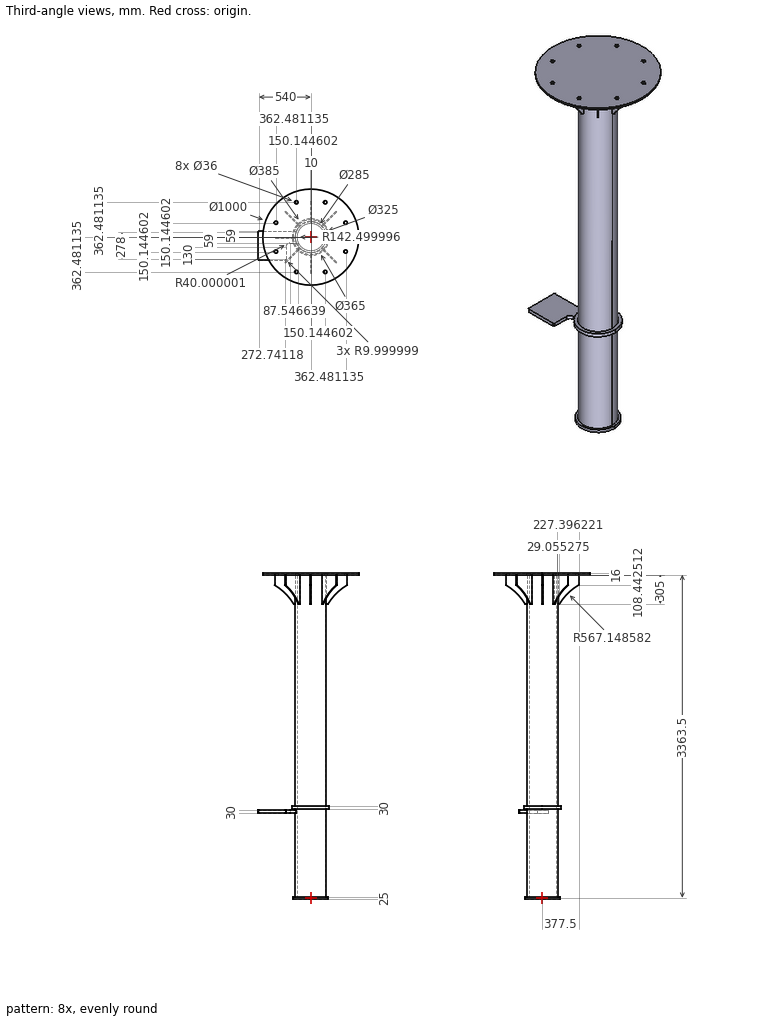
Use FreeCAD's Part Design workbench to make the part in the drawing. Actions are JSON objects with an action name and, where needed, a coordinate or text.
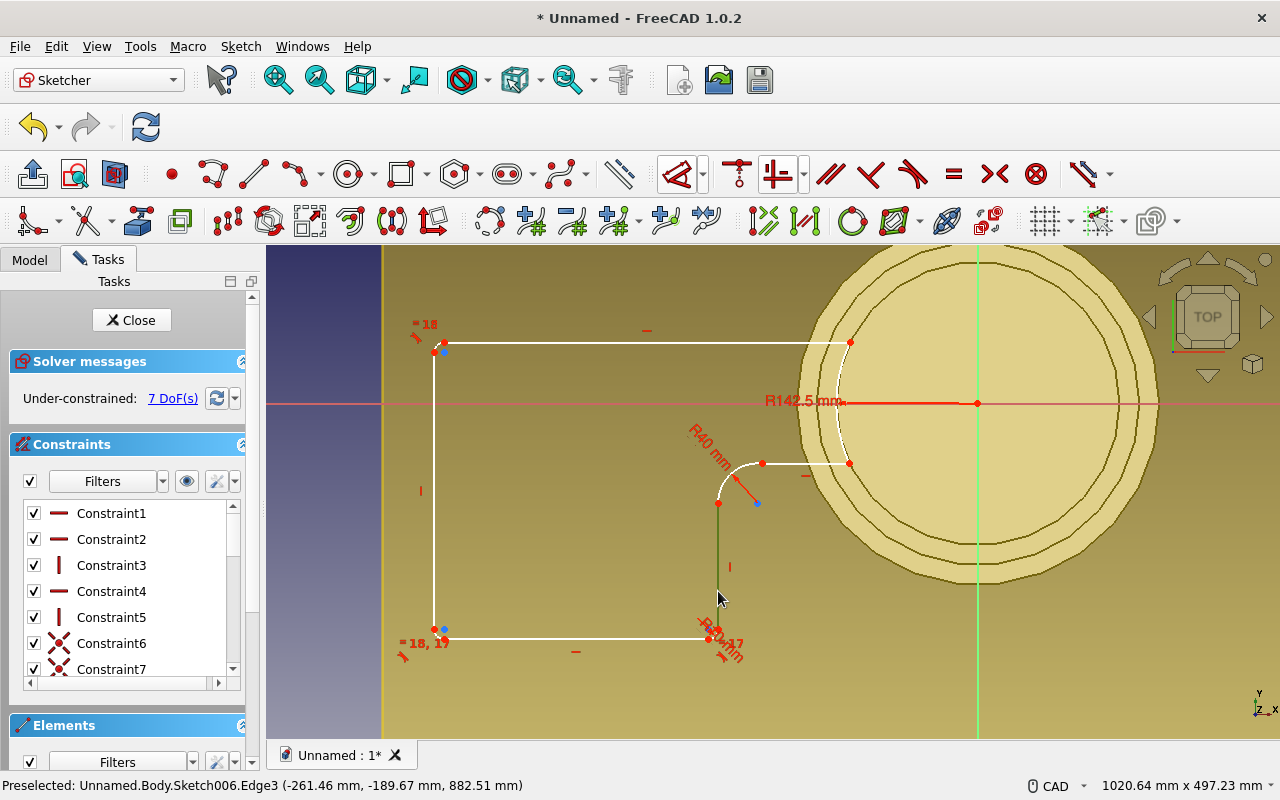
{"action": "key", "text": "i"}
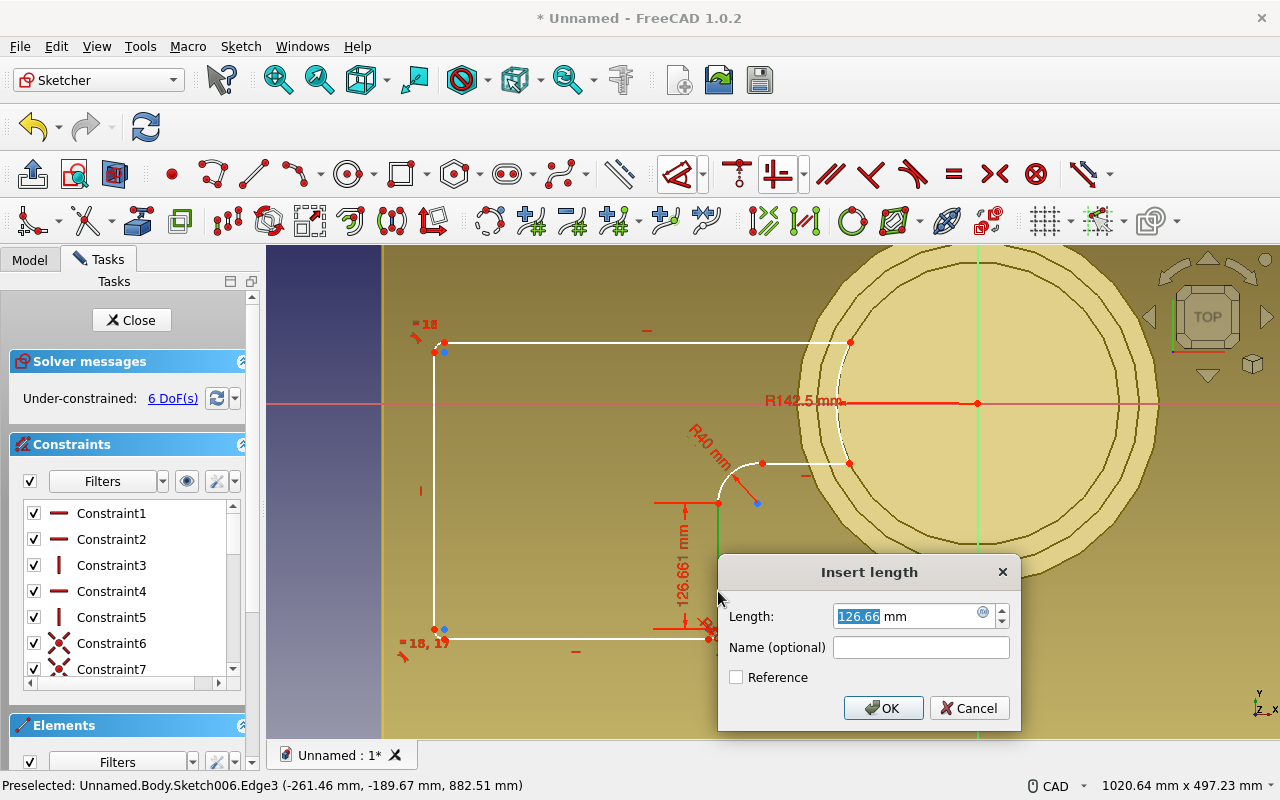
{"action": "type", "text": "130"}
{"action": "key", "text": "Return"}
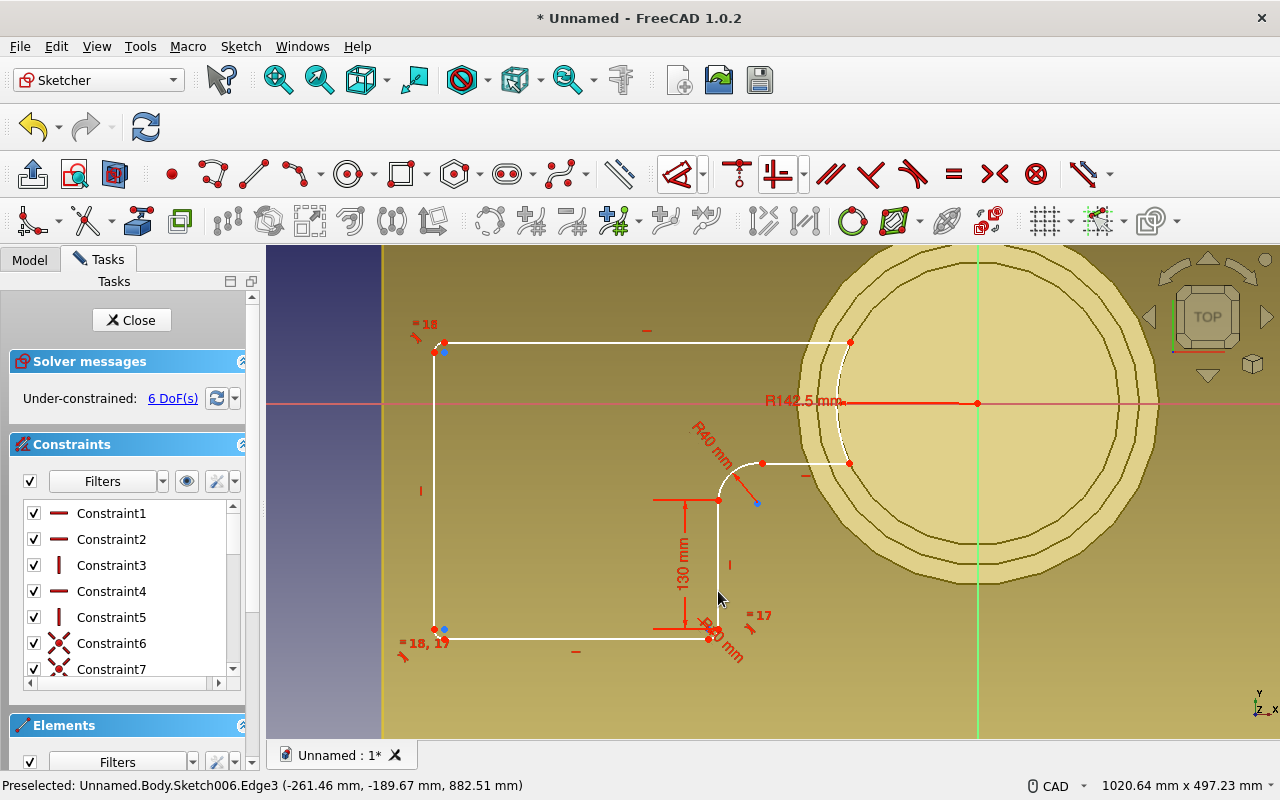
{"action": "left_click", "coordinate": [434, 546]}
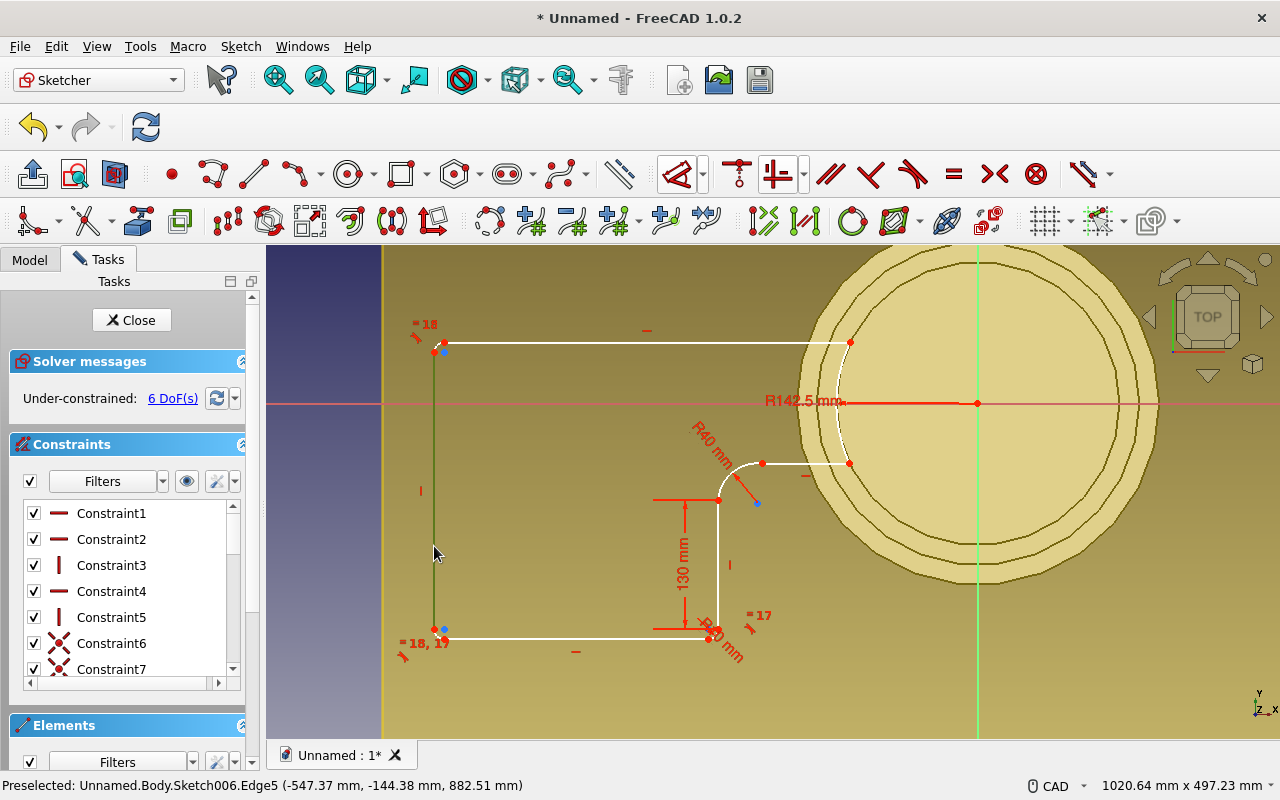
{"action": "left_click", "coordinate": [702, 174]}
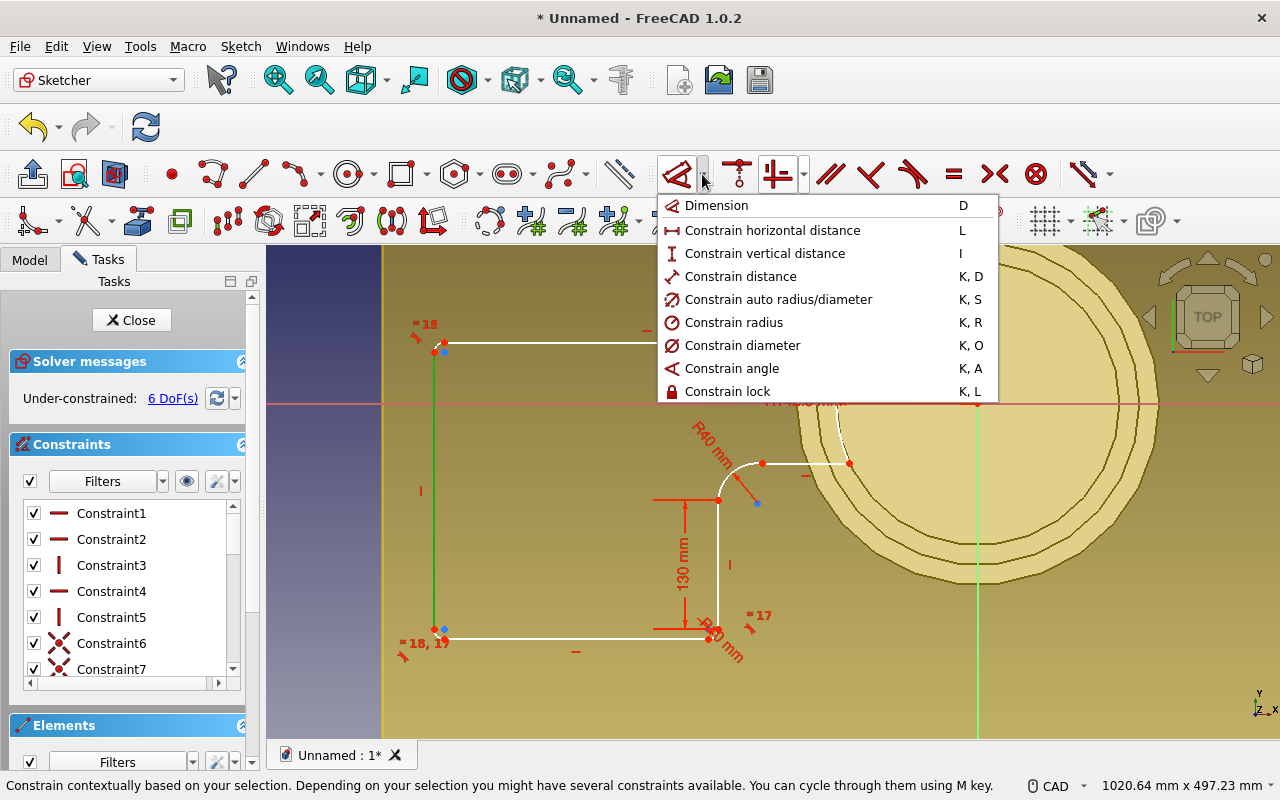
{"action": "left_click", "coordinate": [828, 254]}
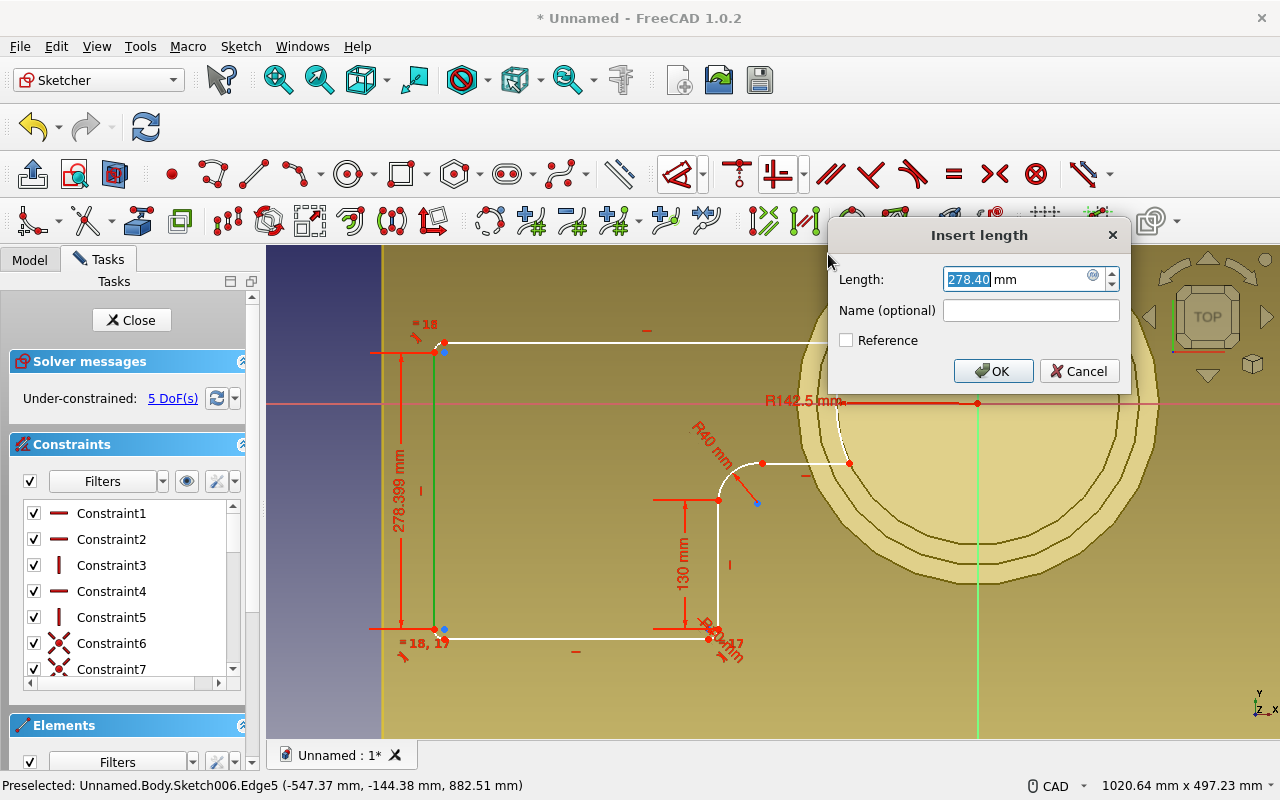
{"action": "type", "text": "278"}
{"action": "key", "text": "Return"}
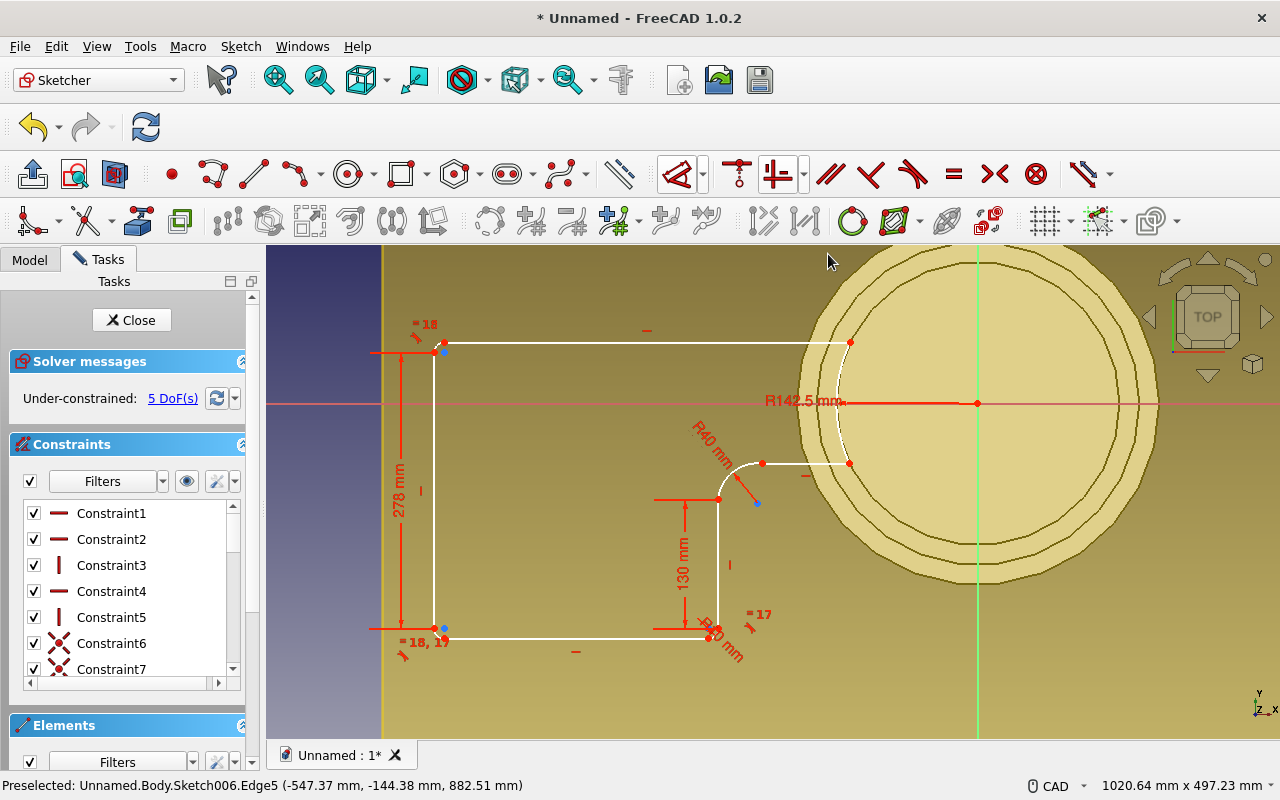
{"action": "scroll", "coordinate": [444, 343], "scroll_direction": "up", "scroll_amount": 2}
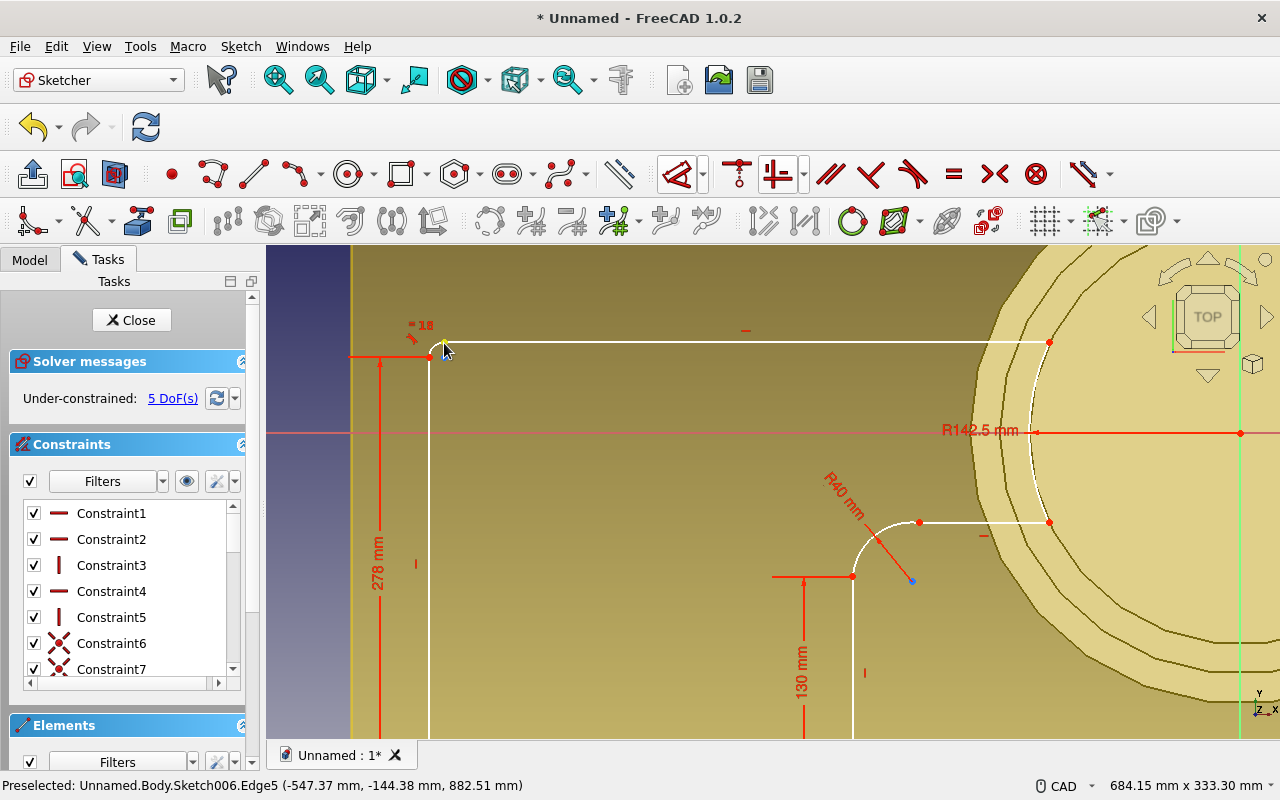
{"action": "left_click", "coordinate": [444, 342]}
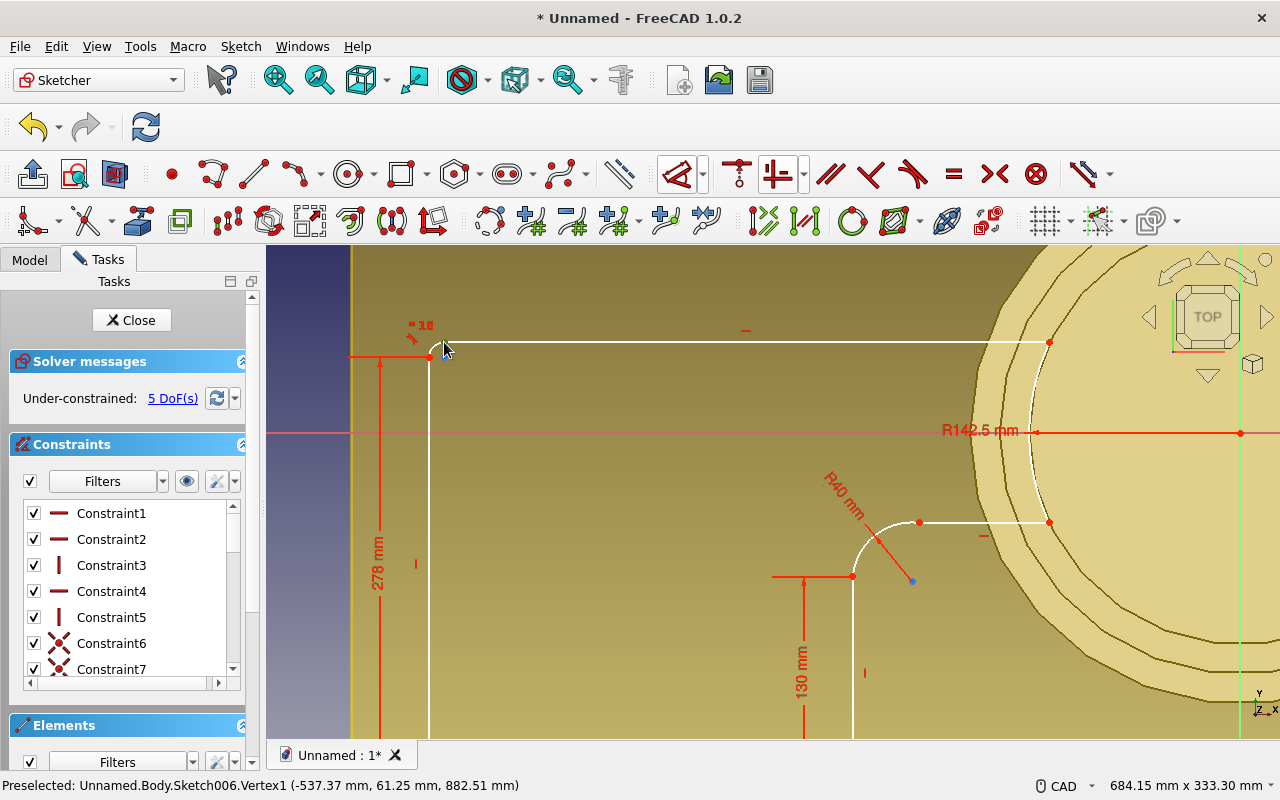
{"action": "key", "text": "i"}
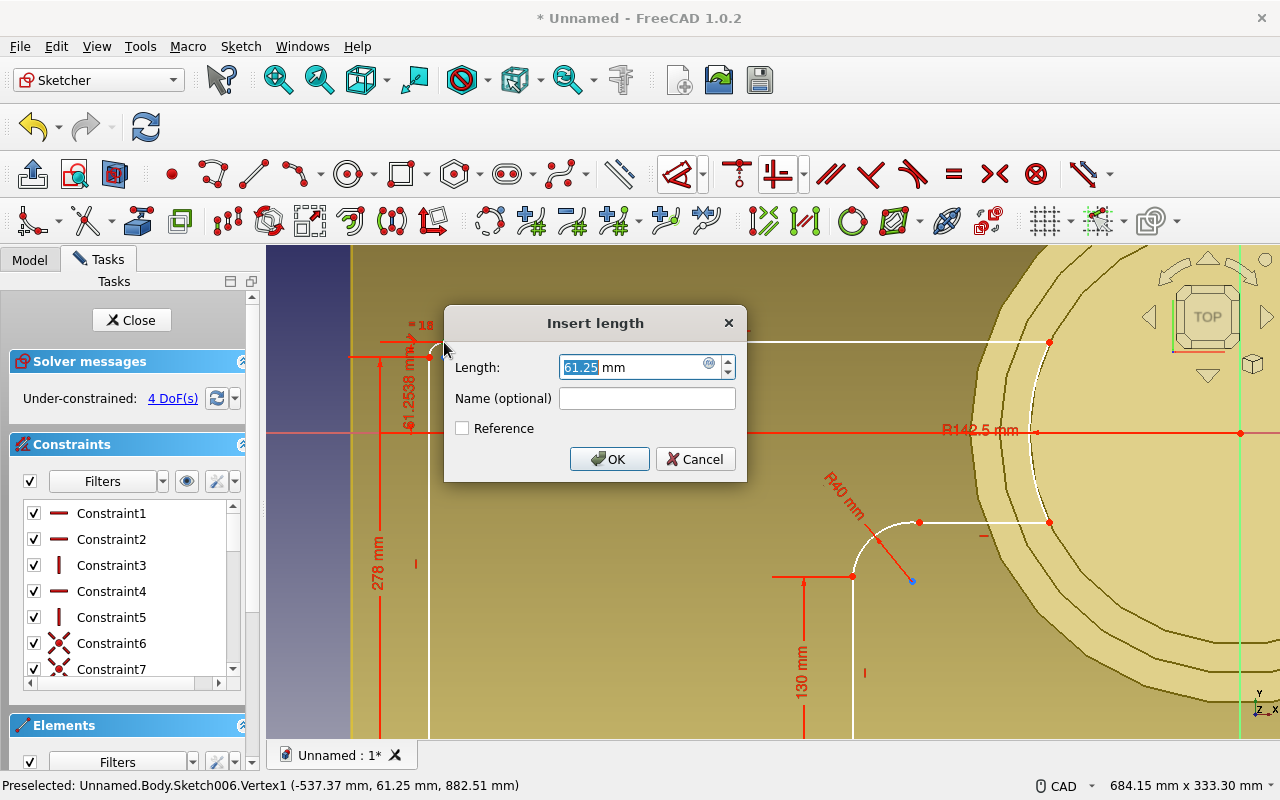
{"action": "type", "text": "59"}
{"action": "key", "text": "Return"}